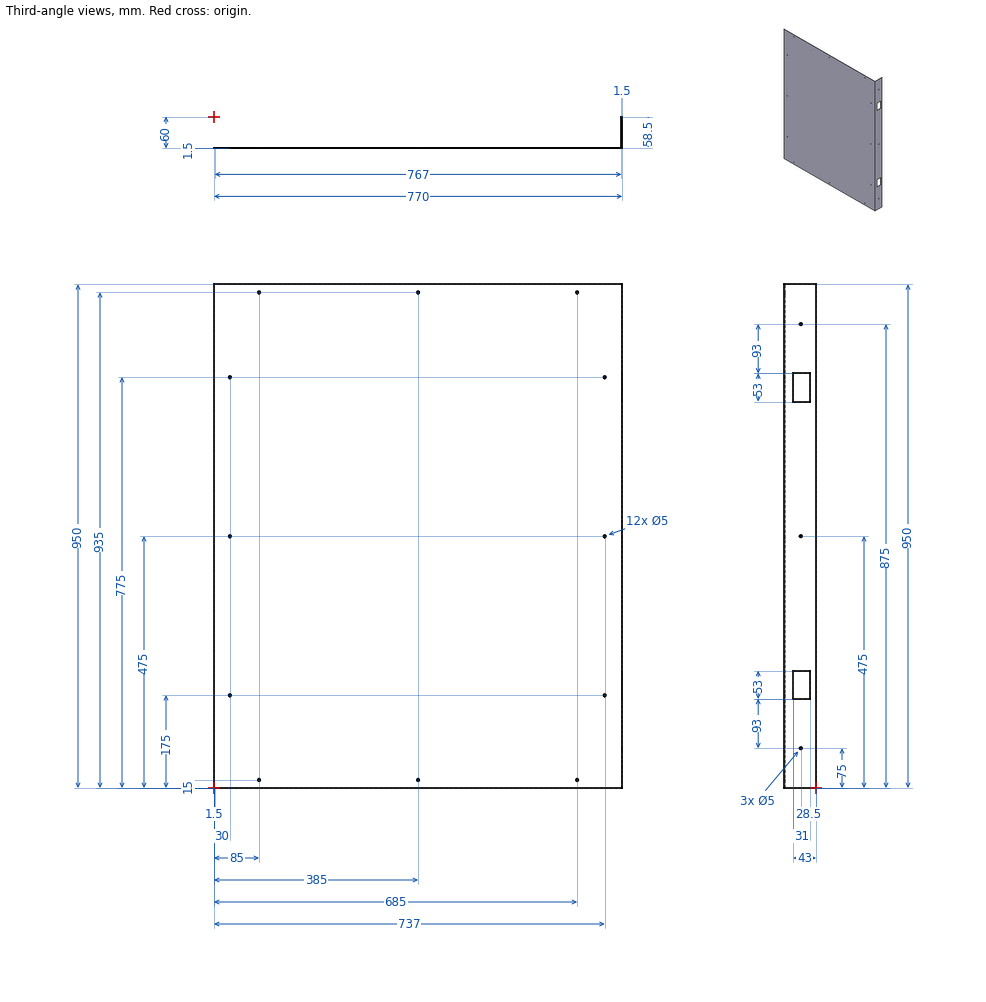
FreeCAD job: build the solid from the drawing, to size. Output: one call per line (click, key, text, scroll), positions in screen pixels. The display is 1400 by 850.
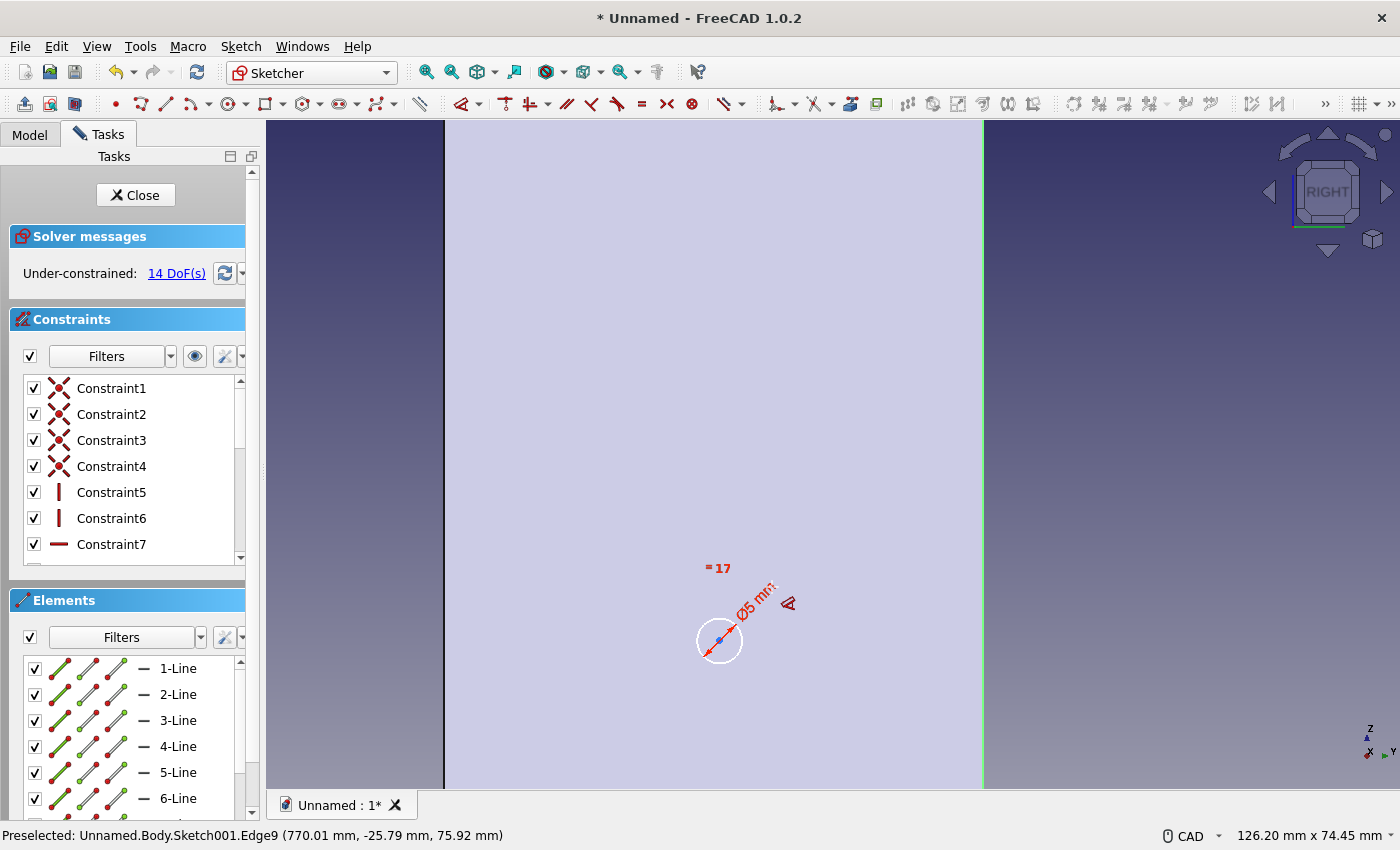
scroll(763, 617, down, 15)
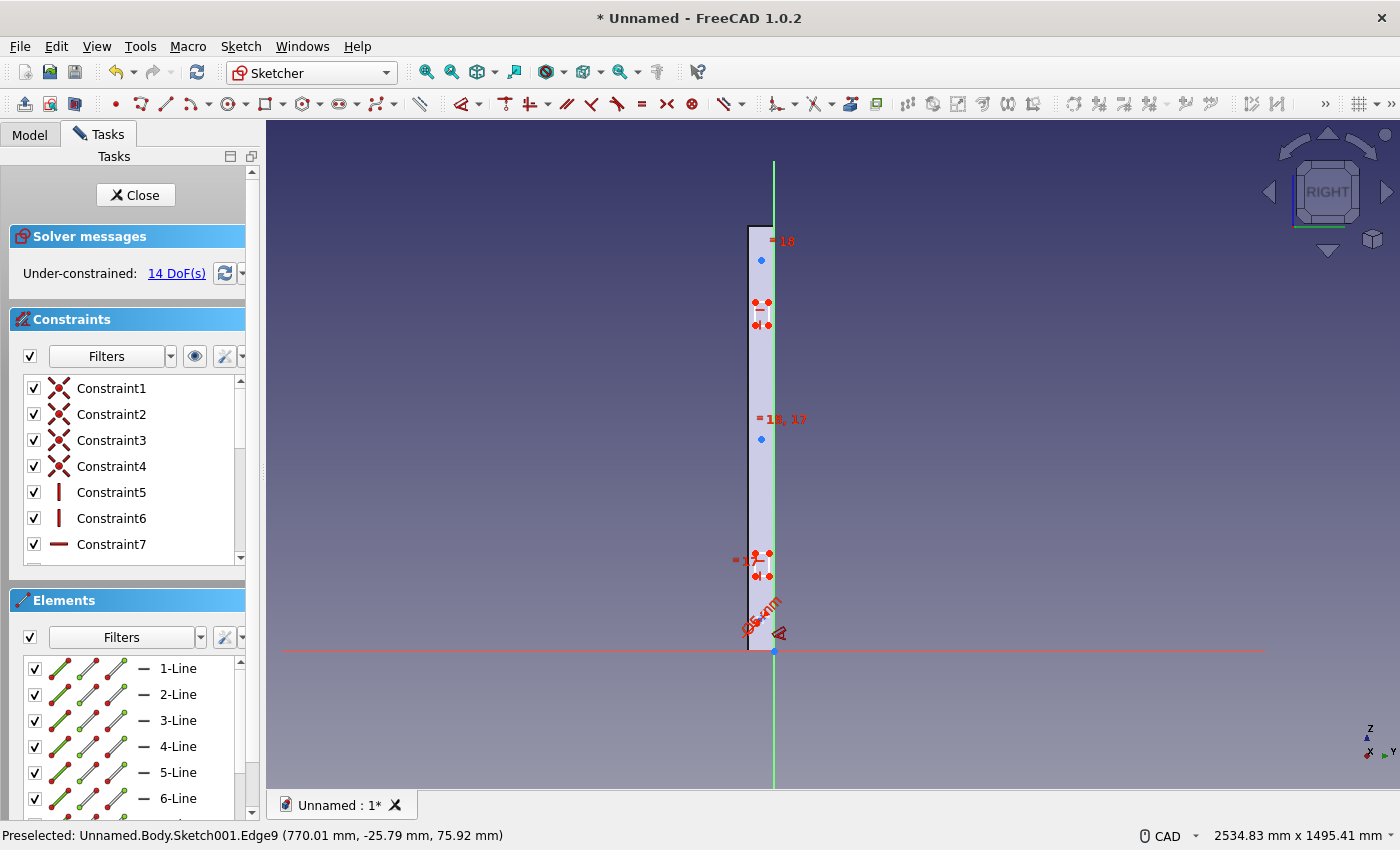
scroll(755, 560, up, 4)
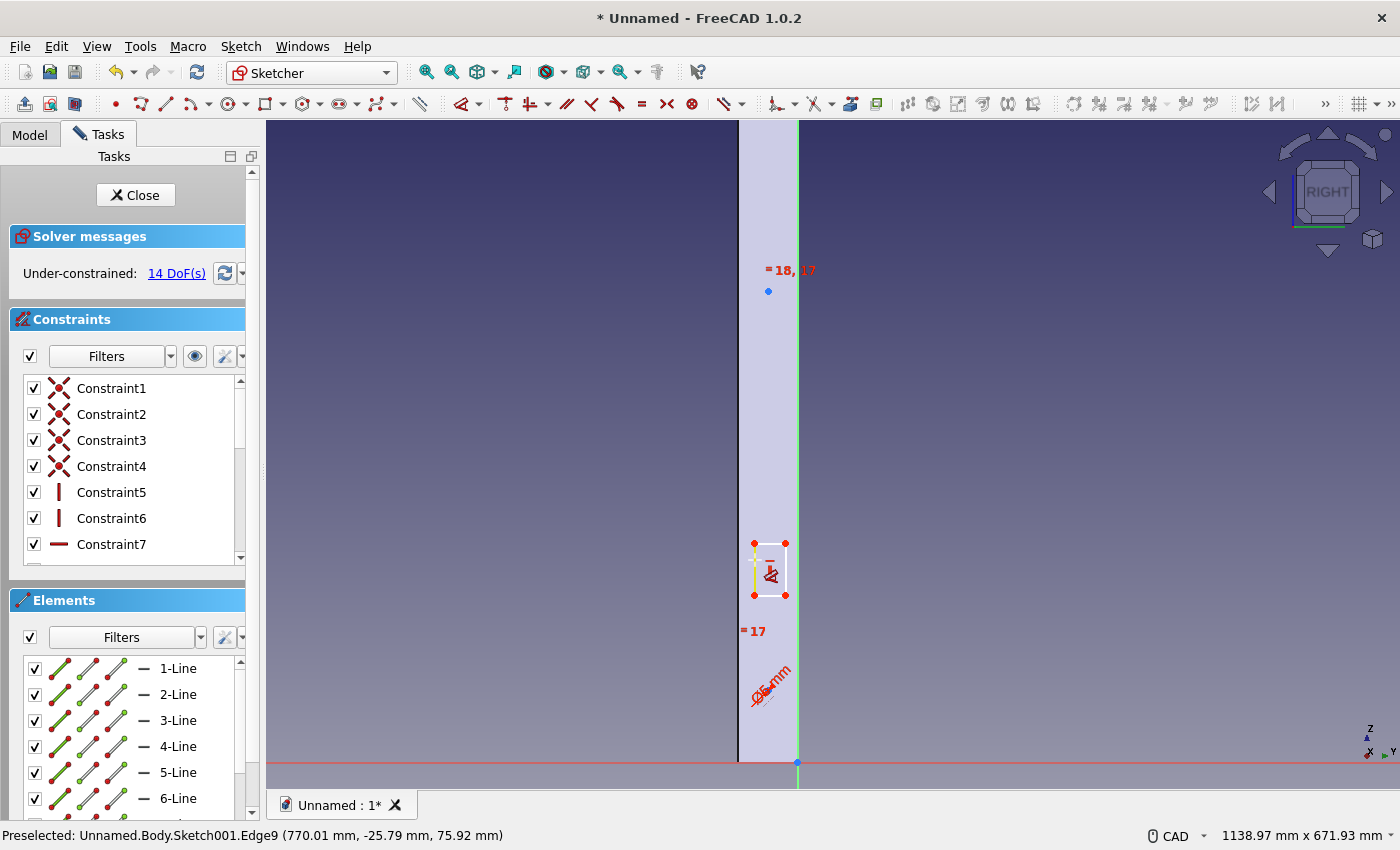
click(755, 559)
click(721, 570)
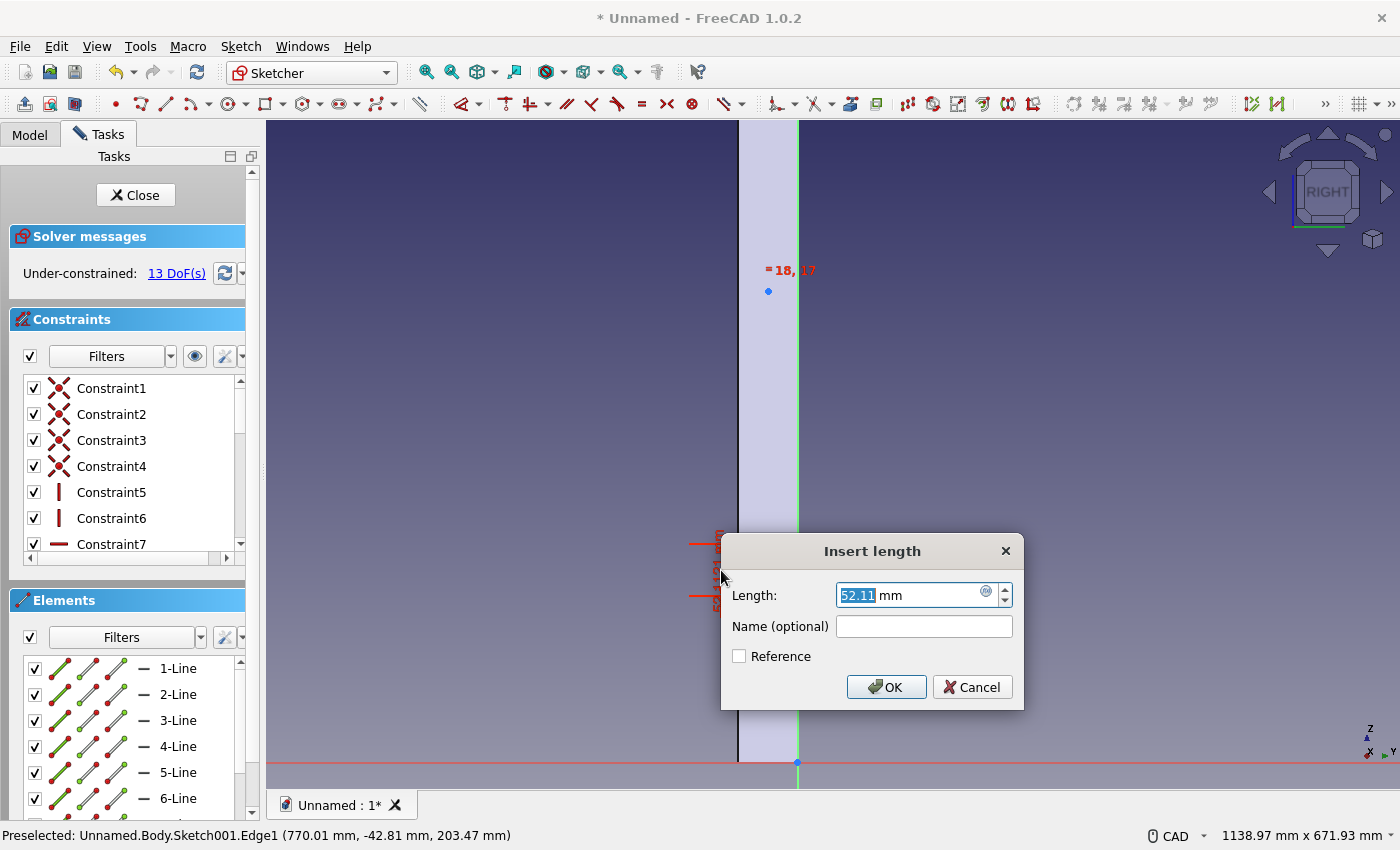
text(53)
key(Return)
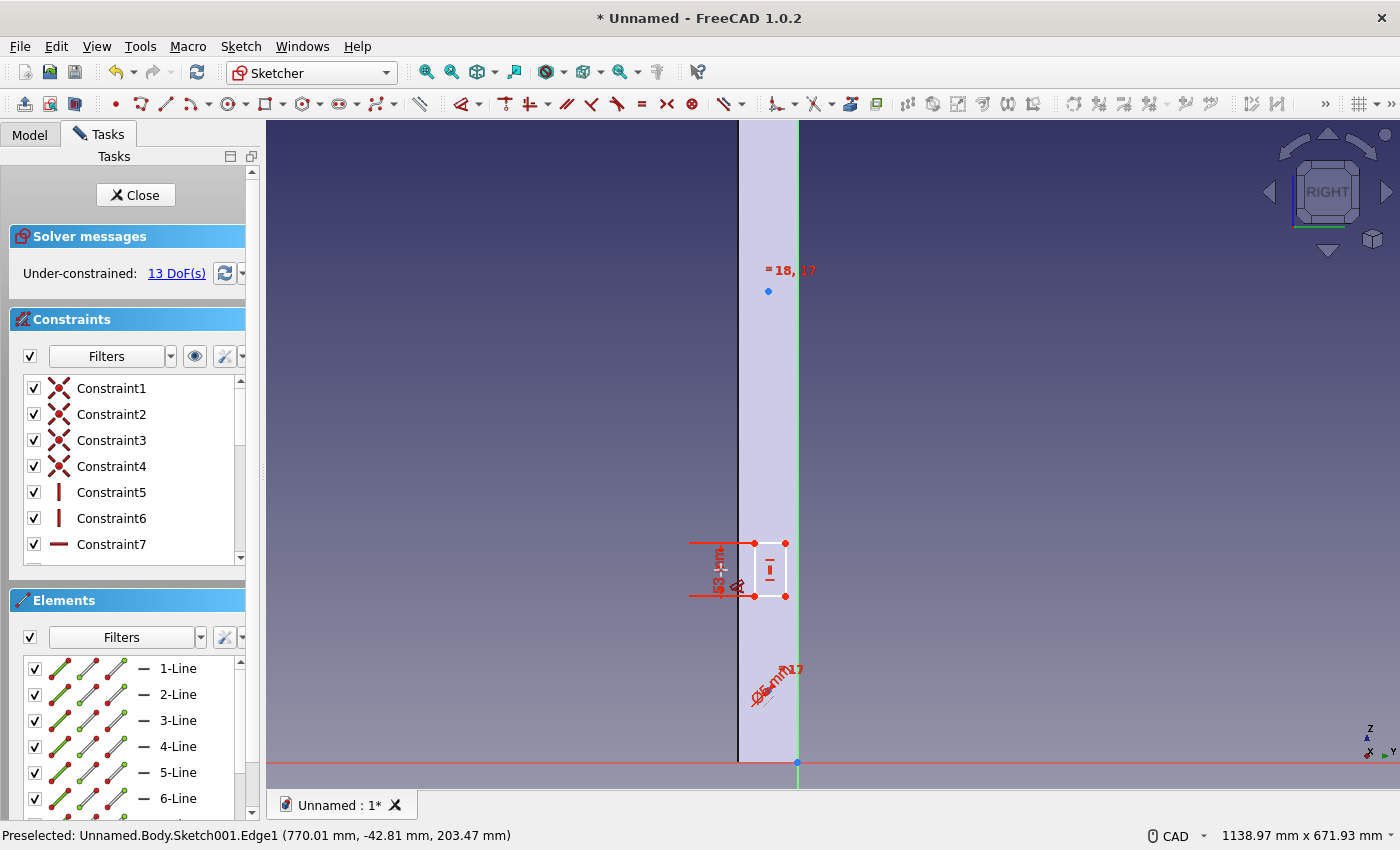
scroll(764, 596, up, 2)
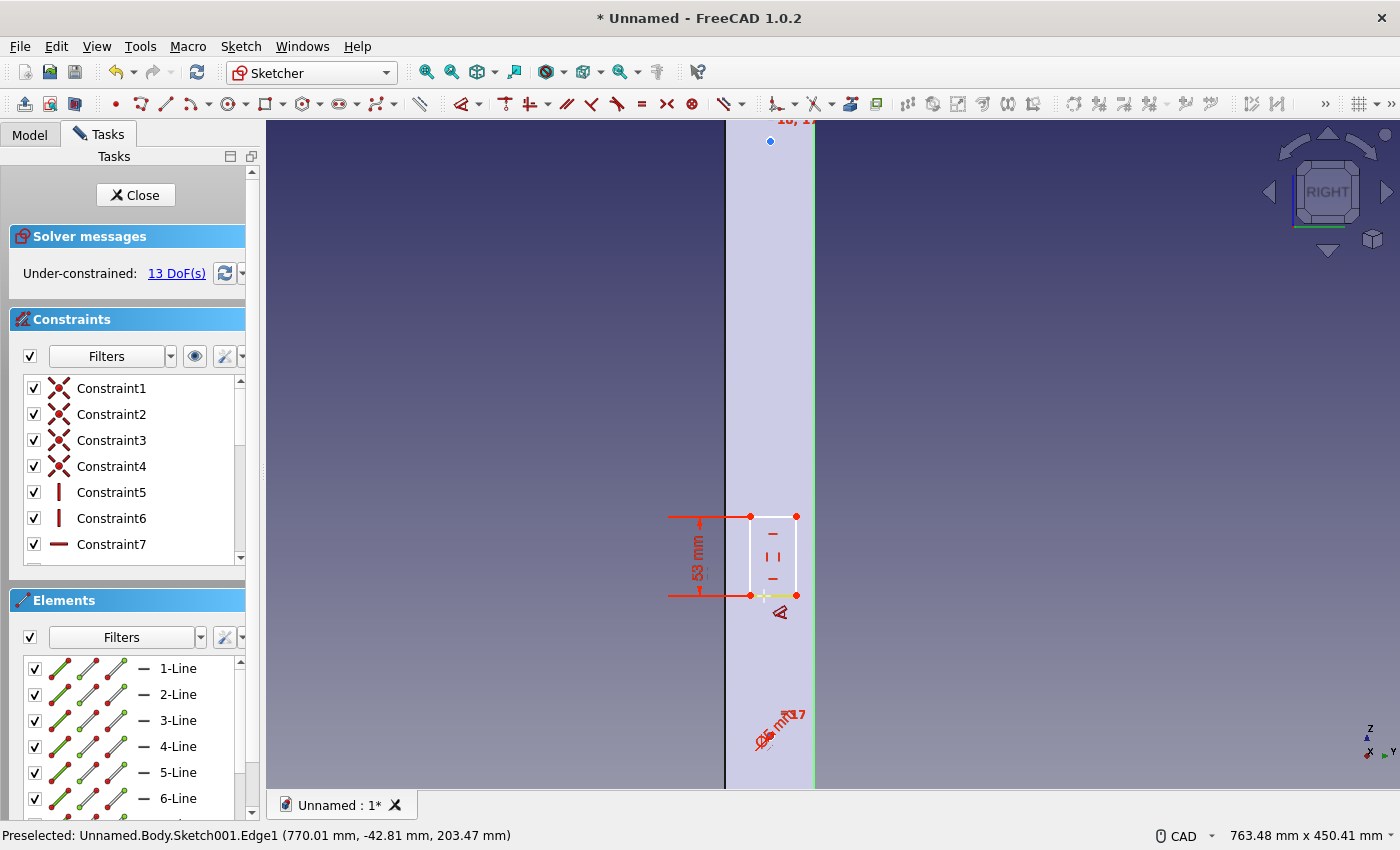
click(764, 596)
click(773, 630)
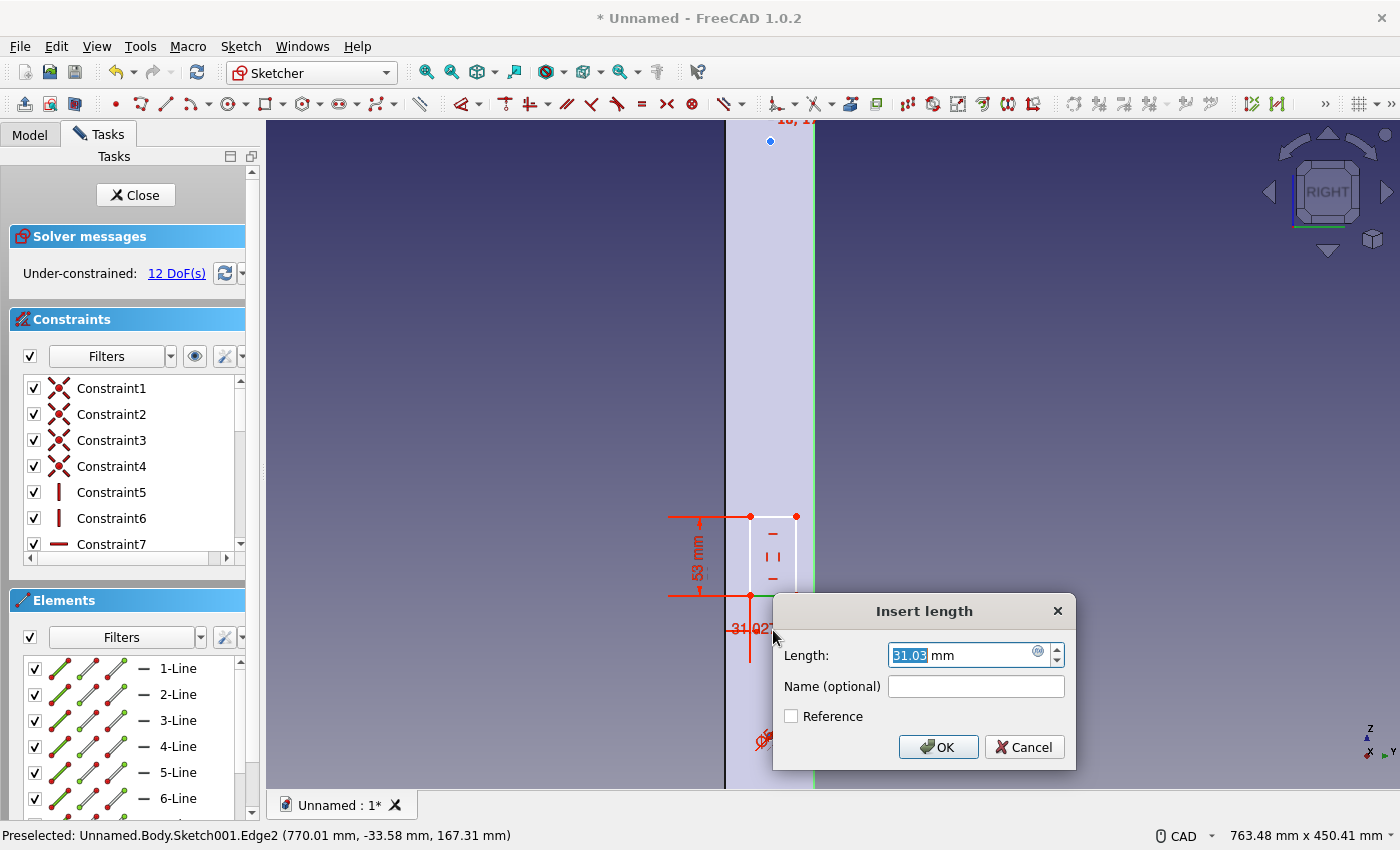
text(31)
key(Return)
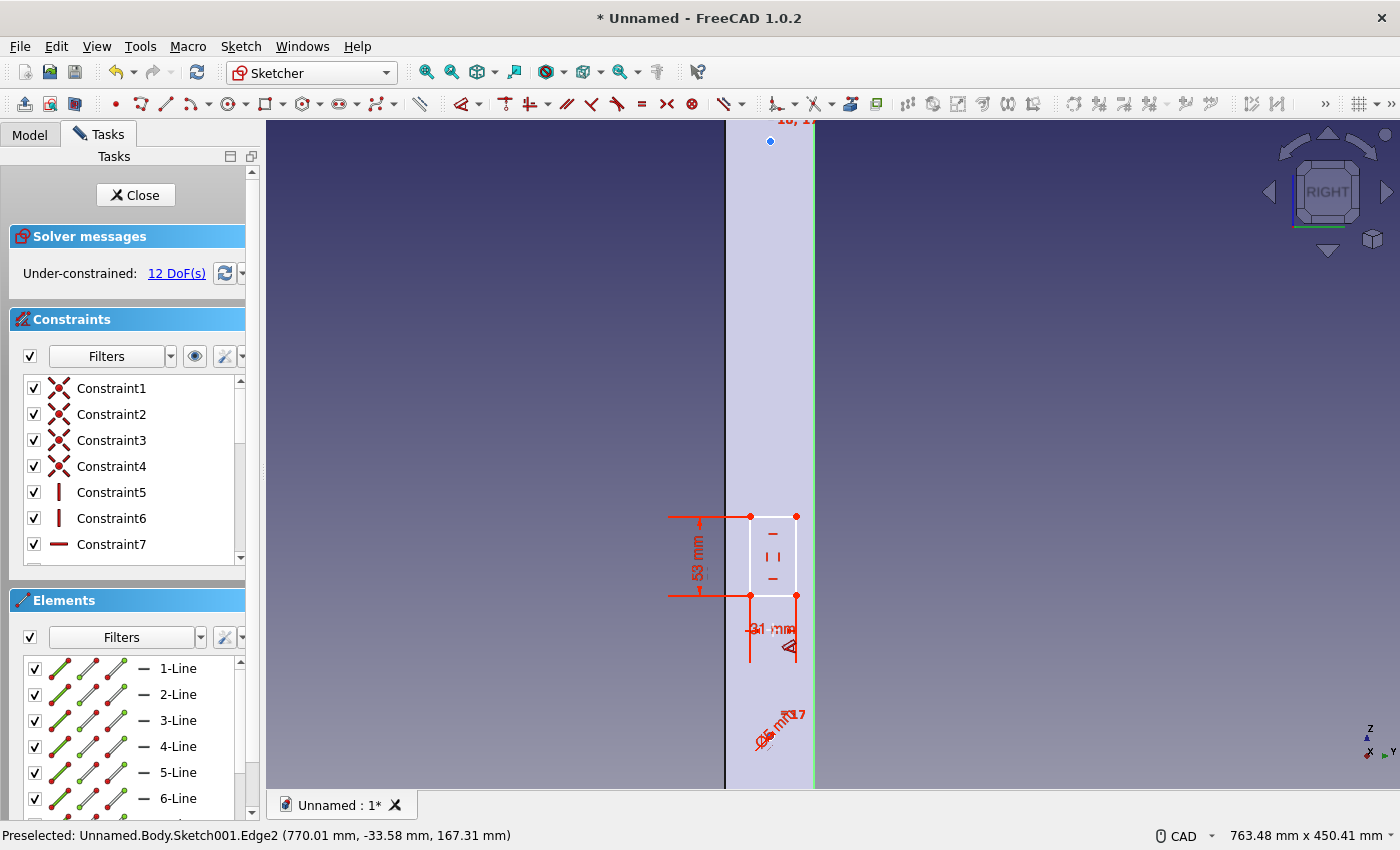
scroll(757, 567, down, 6)